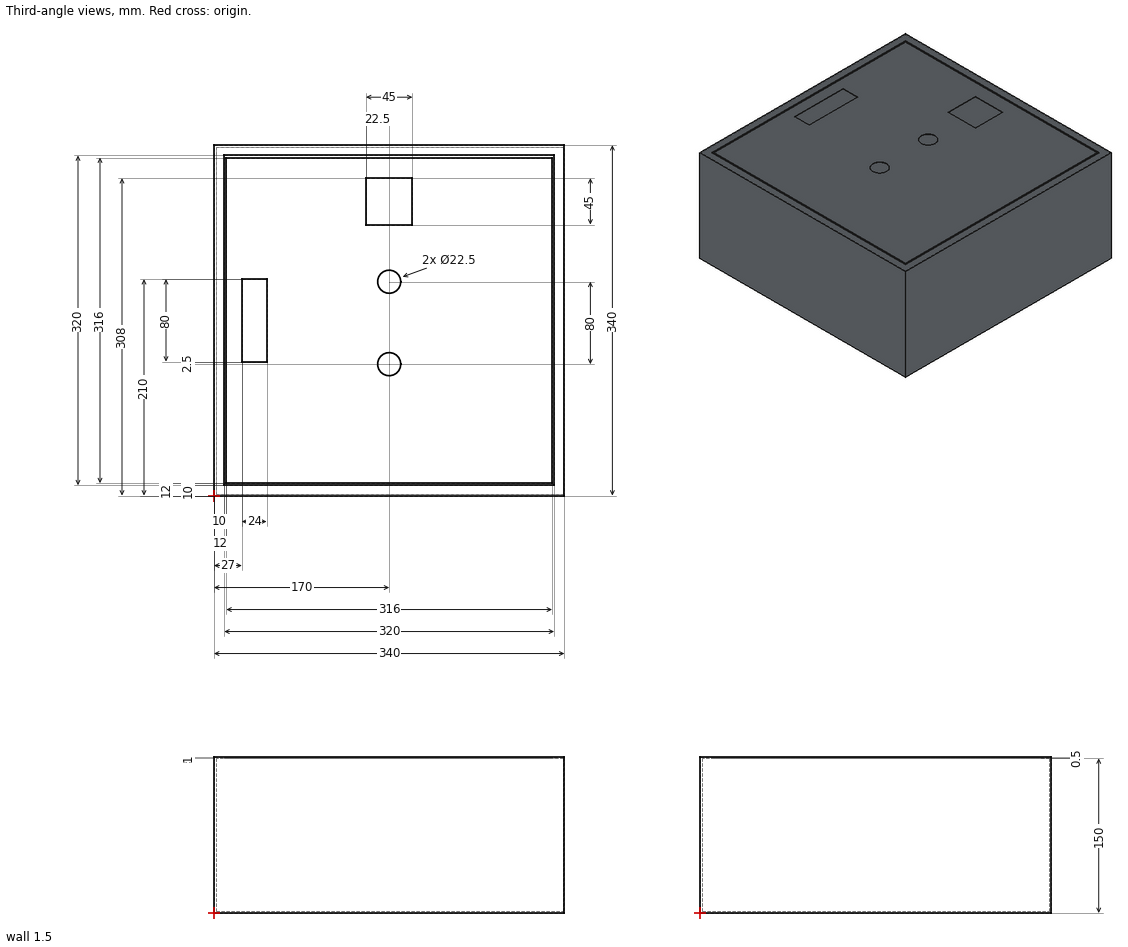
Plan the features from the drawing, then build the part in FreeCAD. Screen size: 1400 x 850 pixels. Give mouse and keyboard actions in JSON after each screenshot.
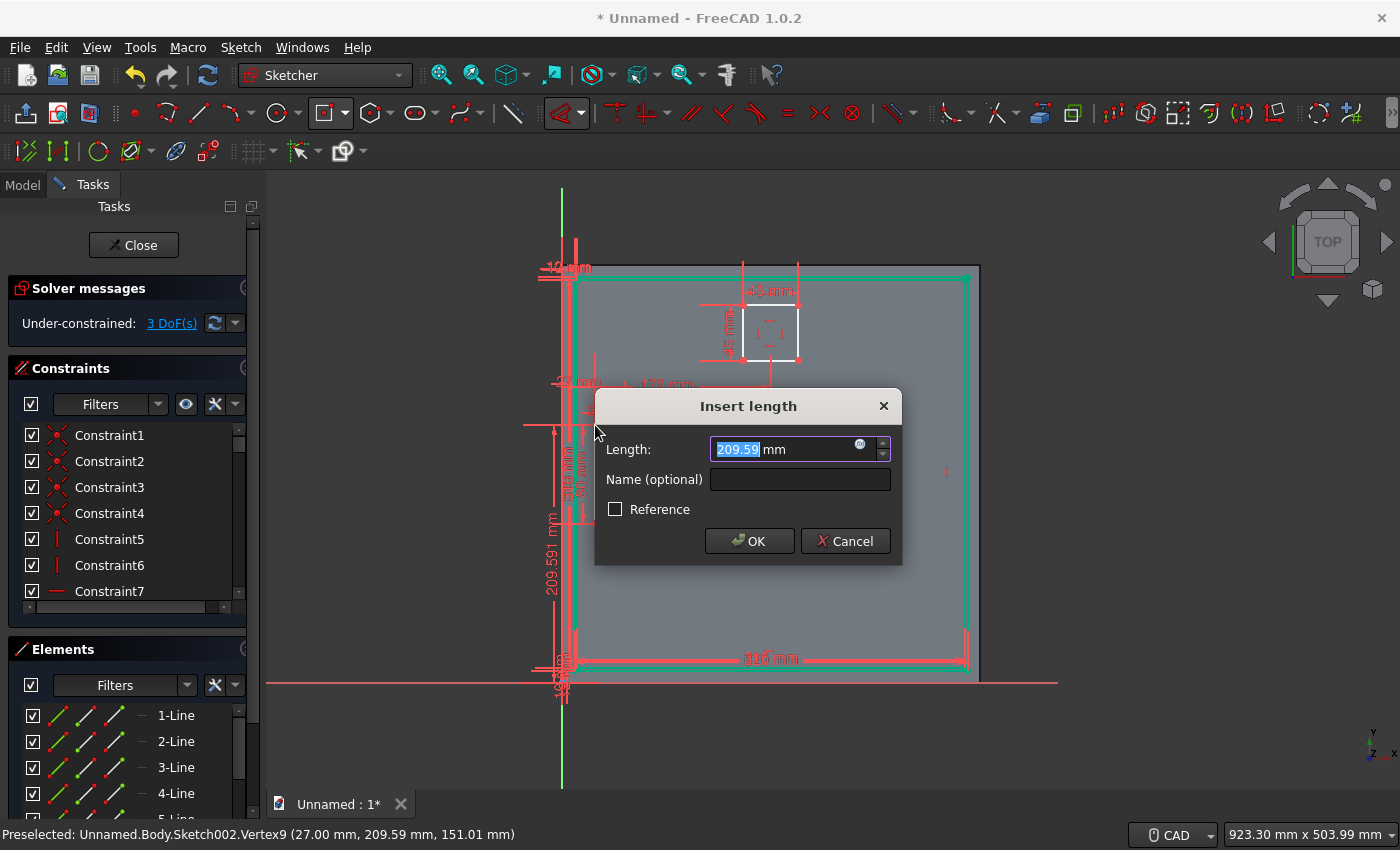
{"action": "type", "text": "210"}
{"action": "key", "text": "Return"}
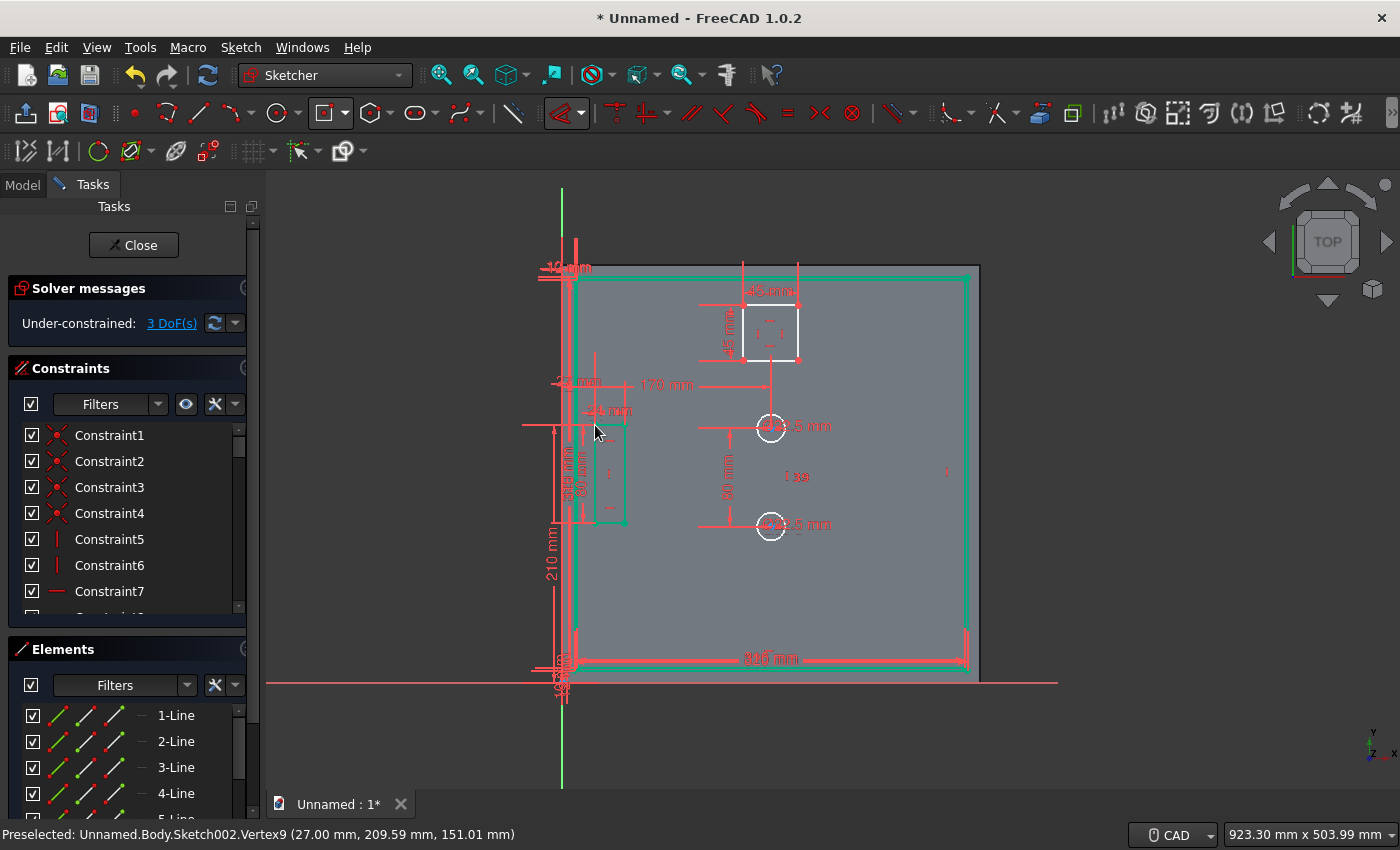
{"action": "left_click", "coordinate": [743, 305]}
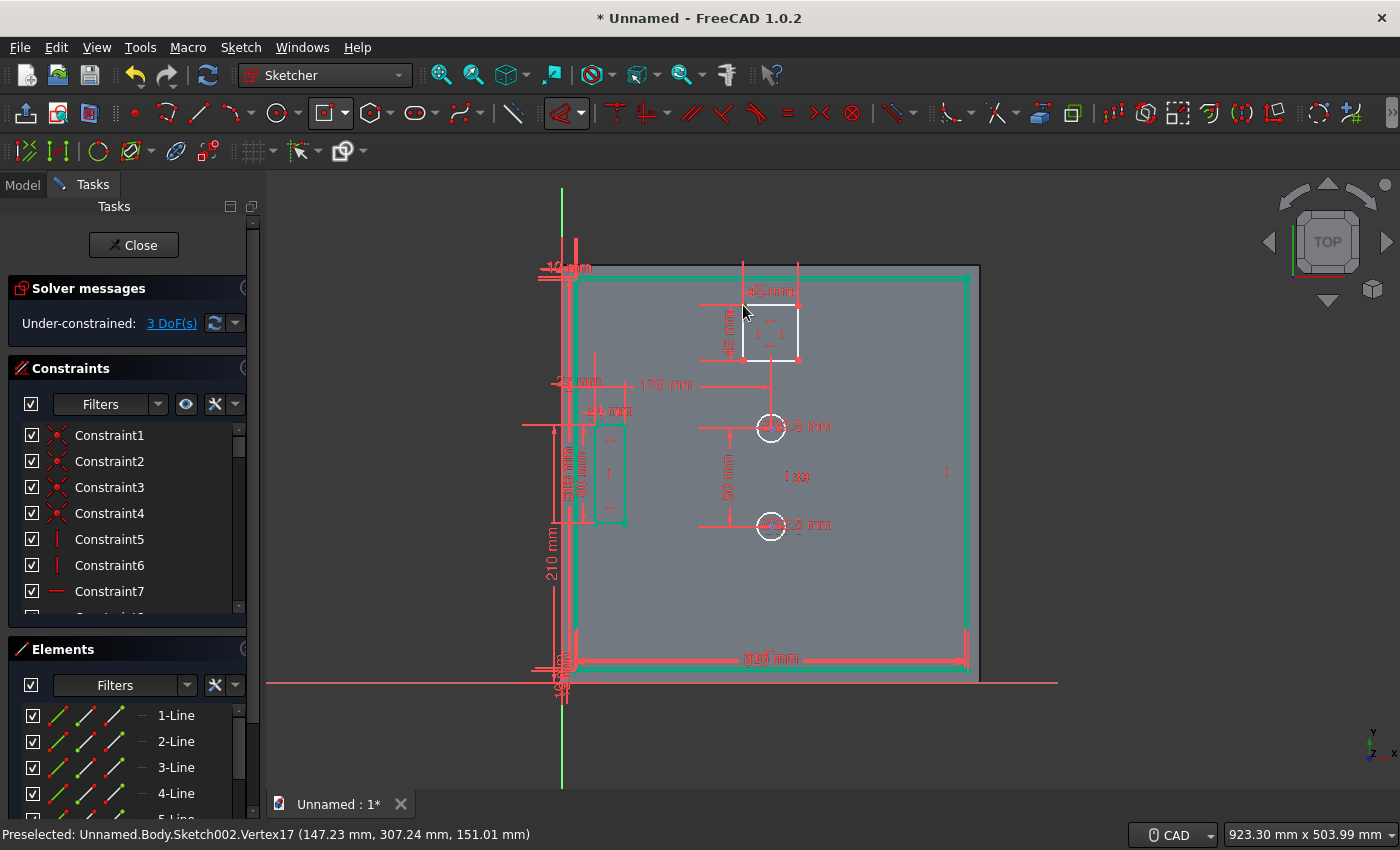
{"action": "key", "text": "i"}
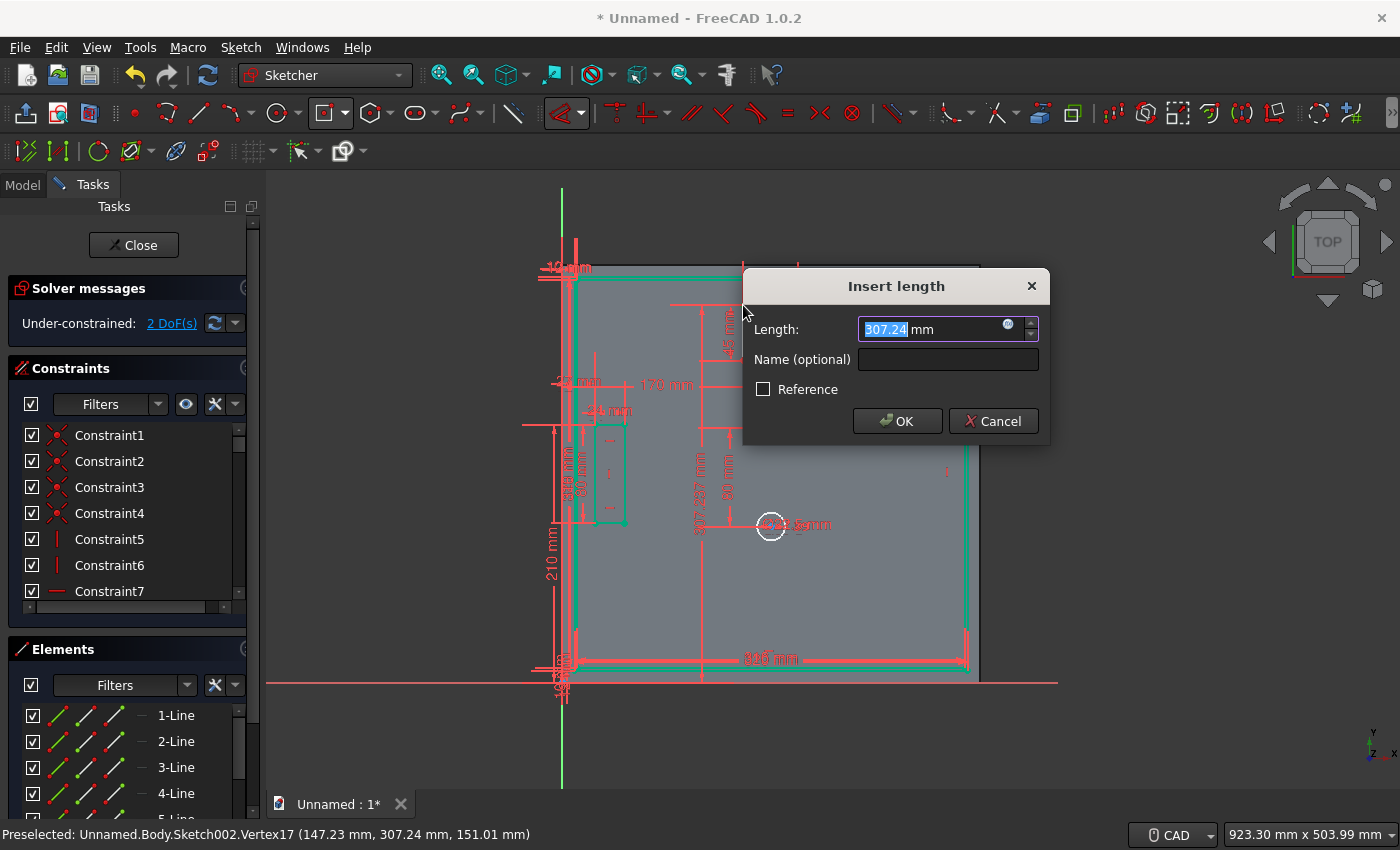
{"action": "type", "text": "308"}
{"action": "key", "text": "Return"}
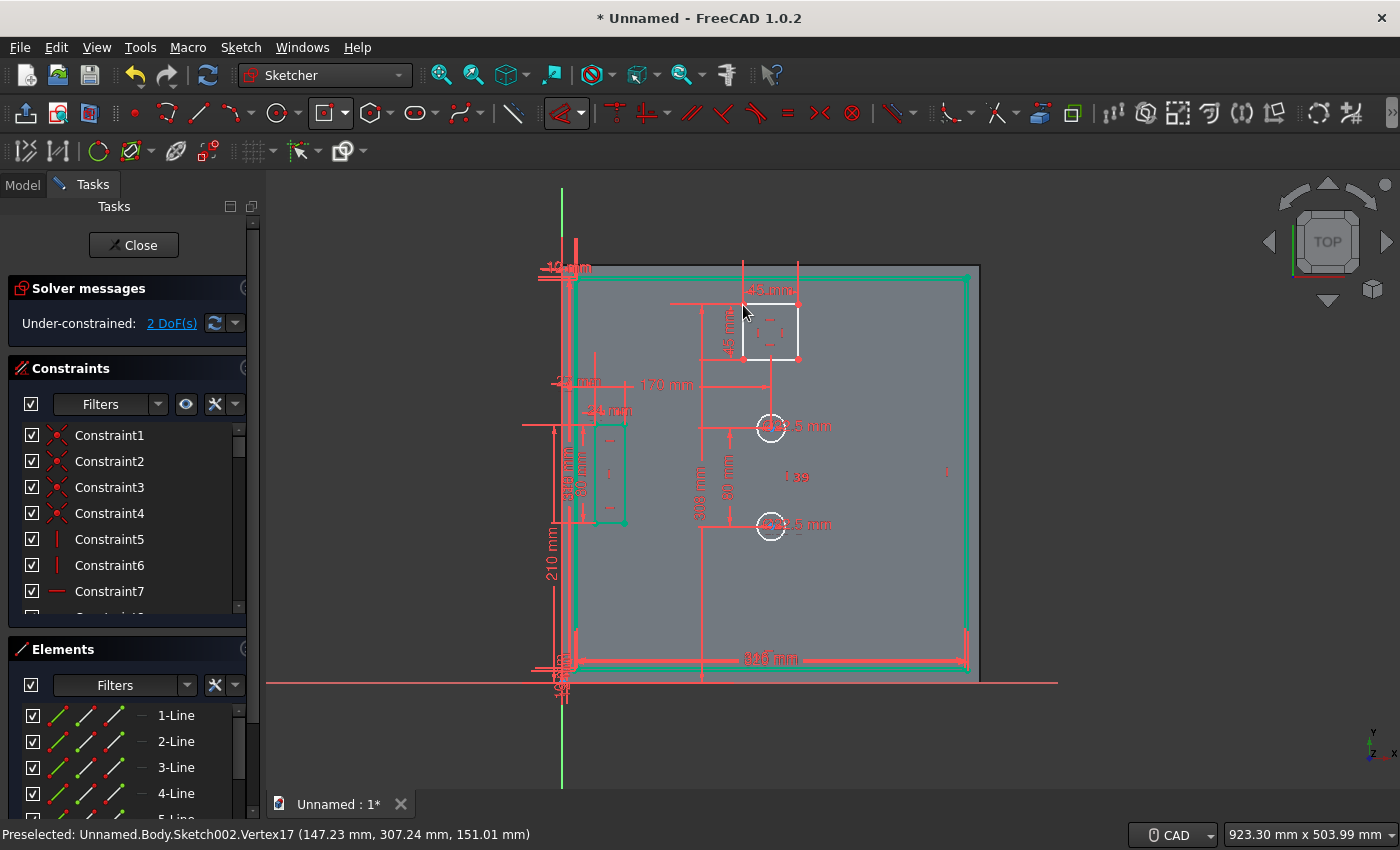
{"action": "scroll", "coordinate": [625, 523], "scroll_direction": "up", "scroll_amount": 13}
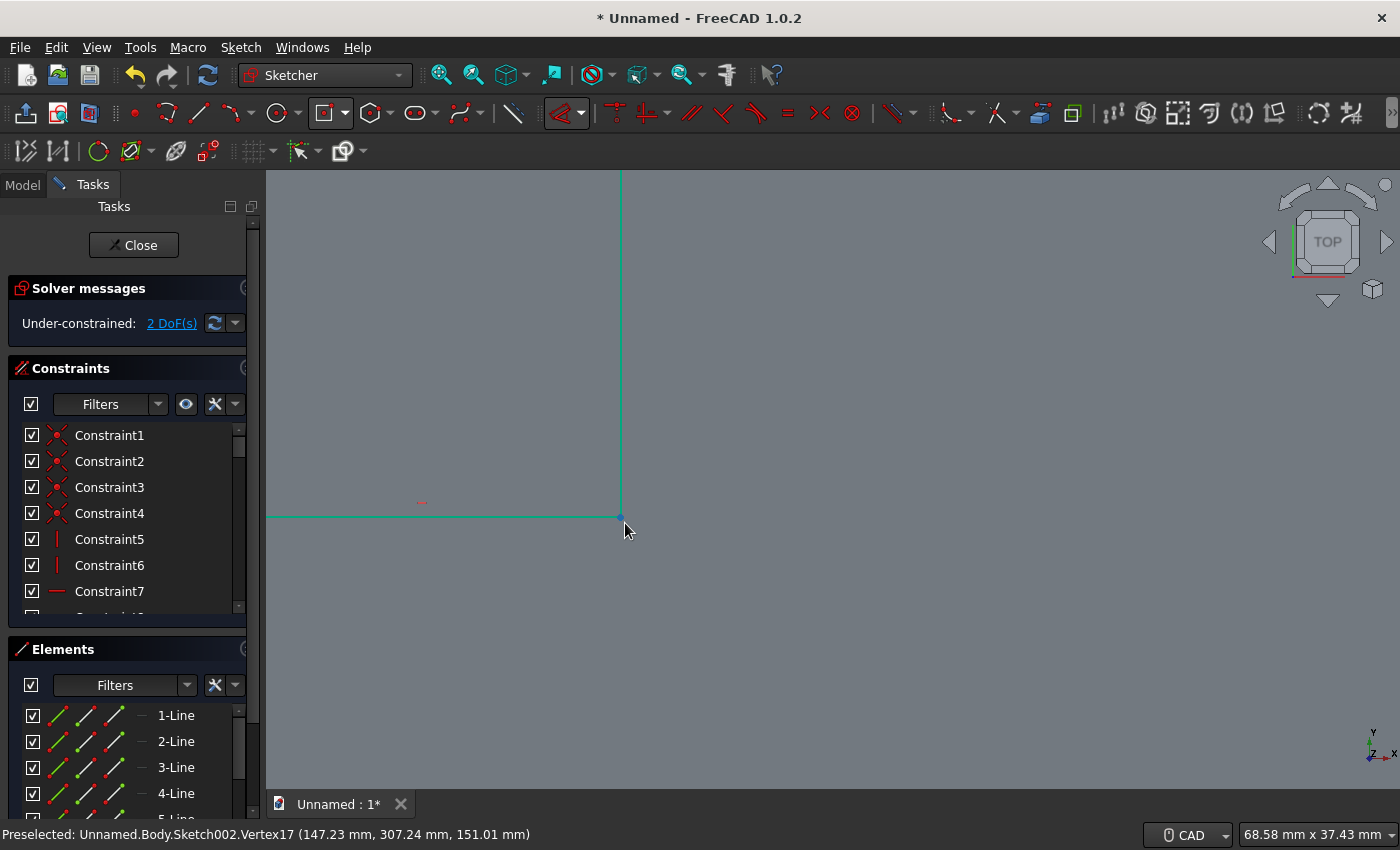
{"action": "left_click", "coordinate": [621, 517]}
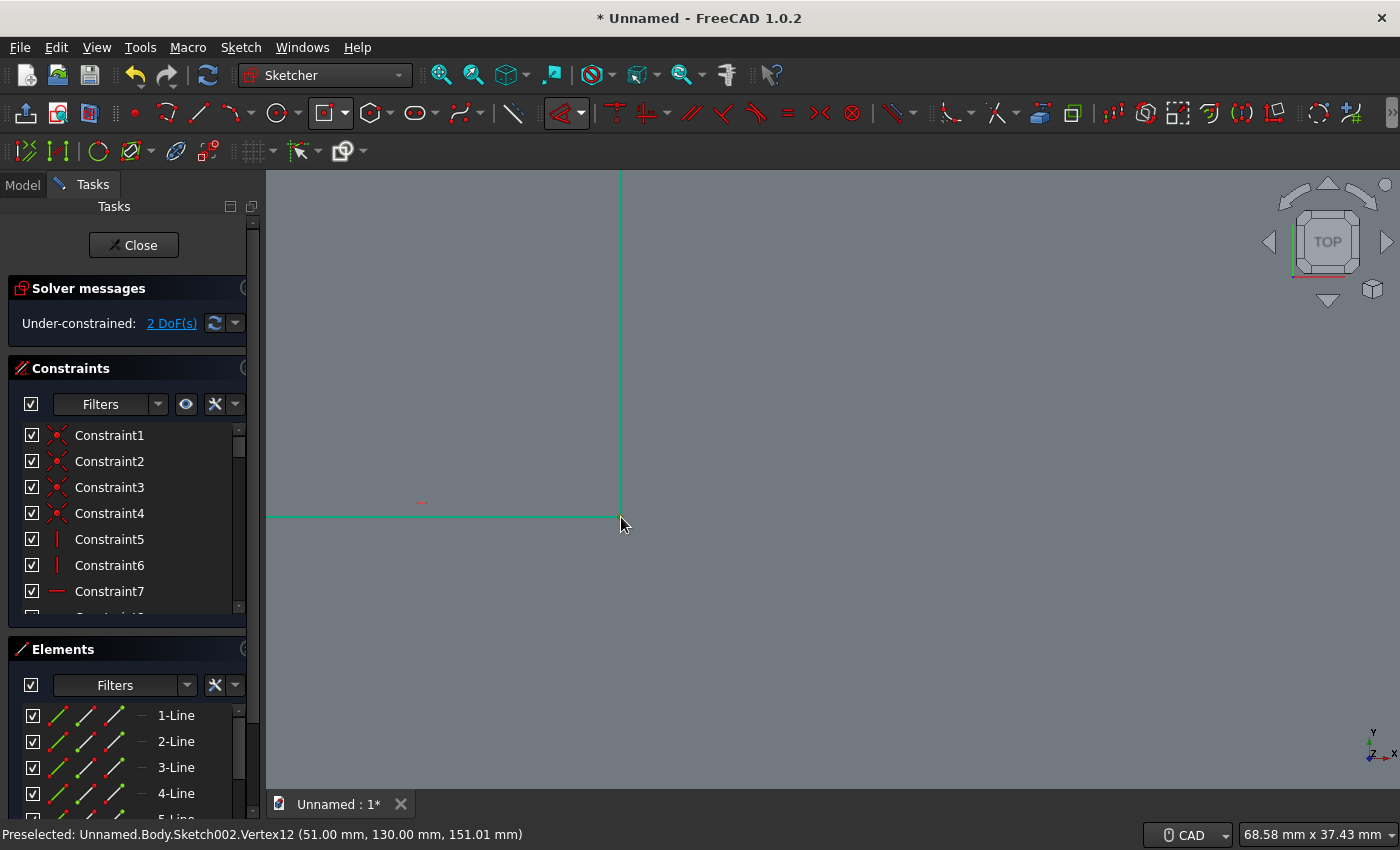
{"action": "scroll", "coordinate": [625, 523], "scroll_direction": "down", "scroll_amount": 13}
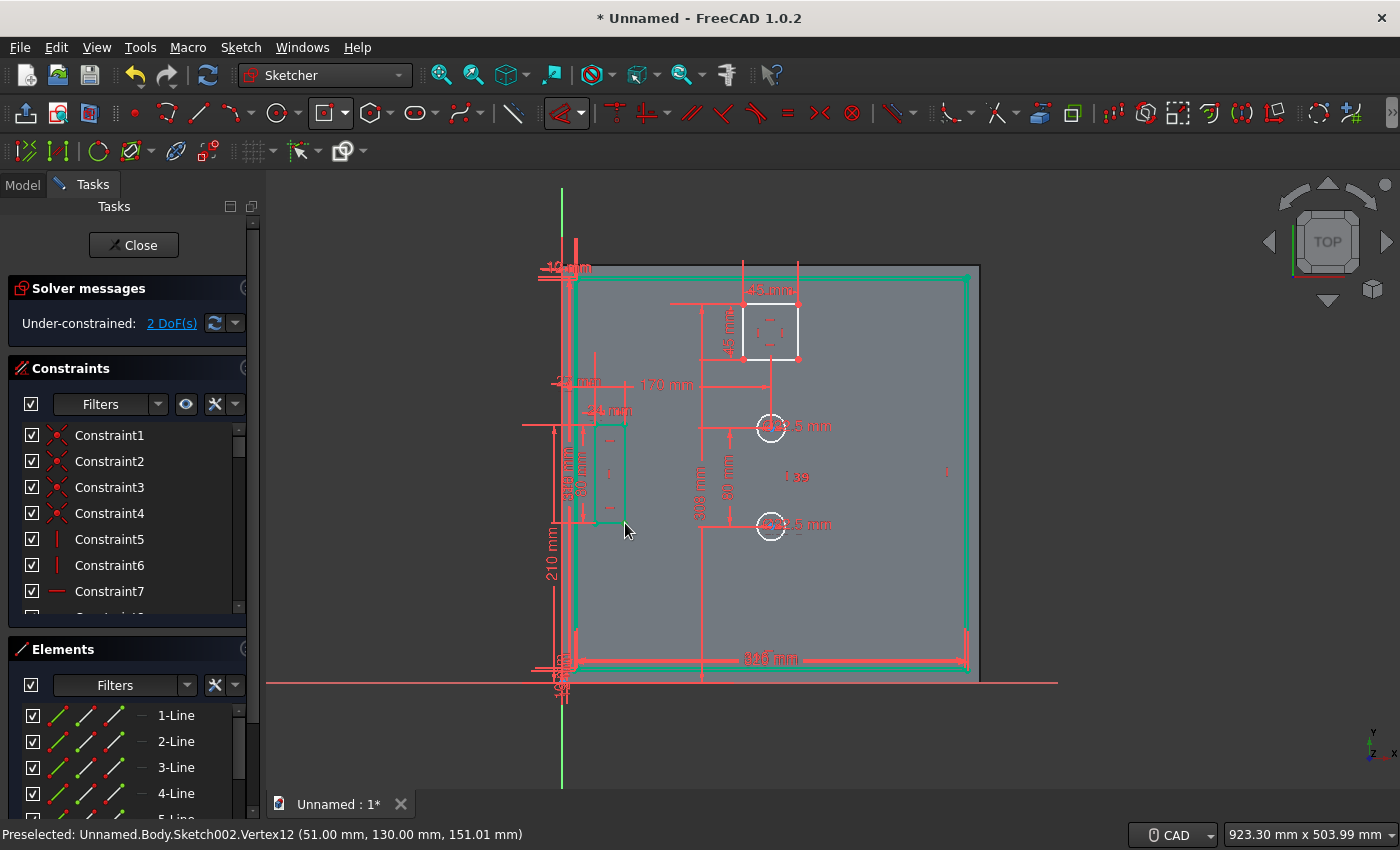
{"action": "scroll", "coordinate": [771, 527], "scroll_direction": "up", "scroll_amount": 13}